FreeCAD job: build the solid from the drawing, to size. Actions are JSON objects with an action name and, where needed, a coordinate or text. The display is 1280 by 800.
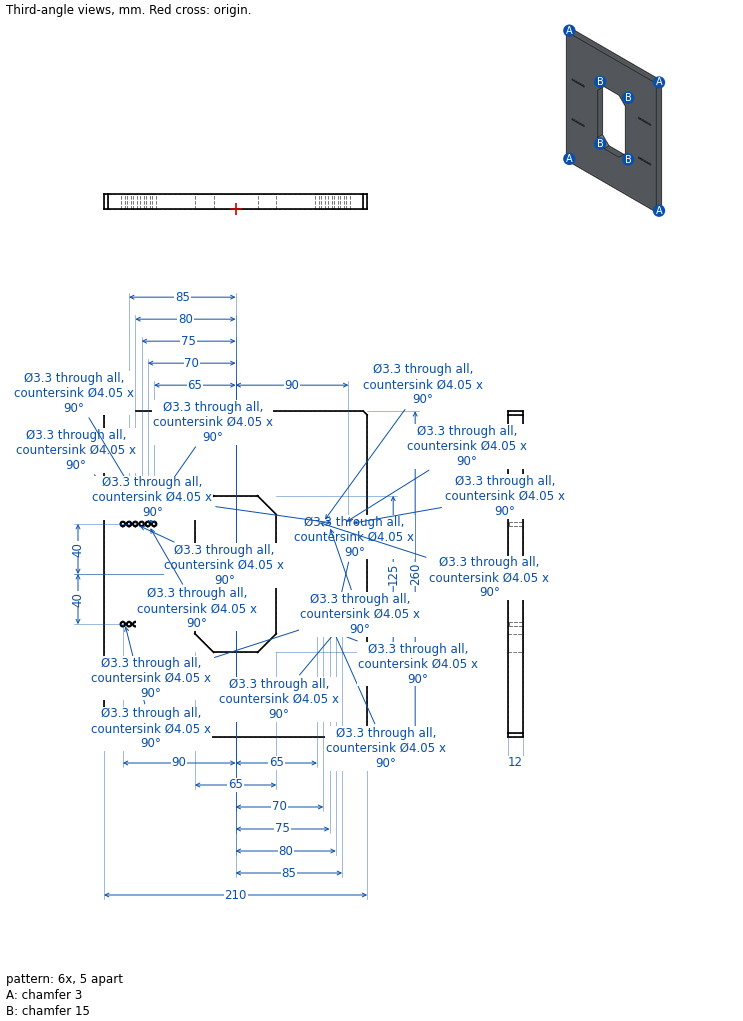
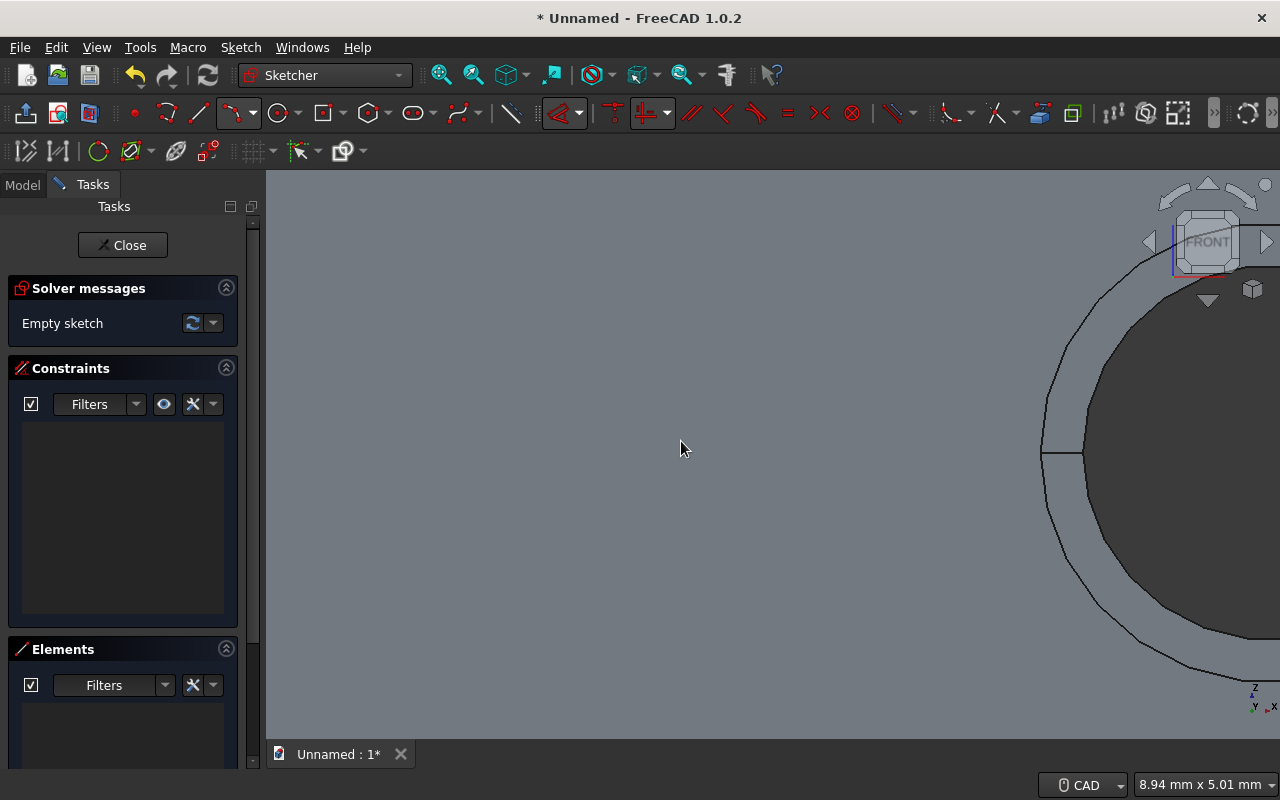
{"action": "left_click", "coordinate": [278, 114]}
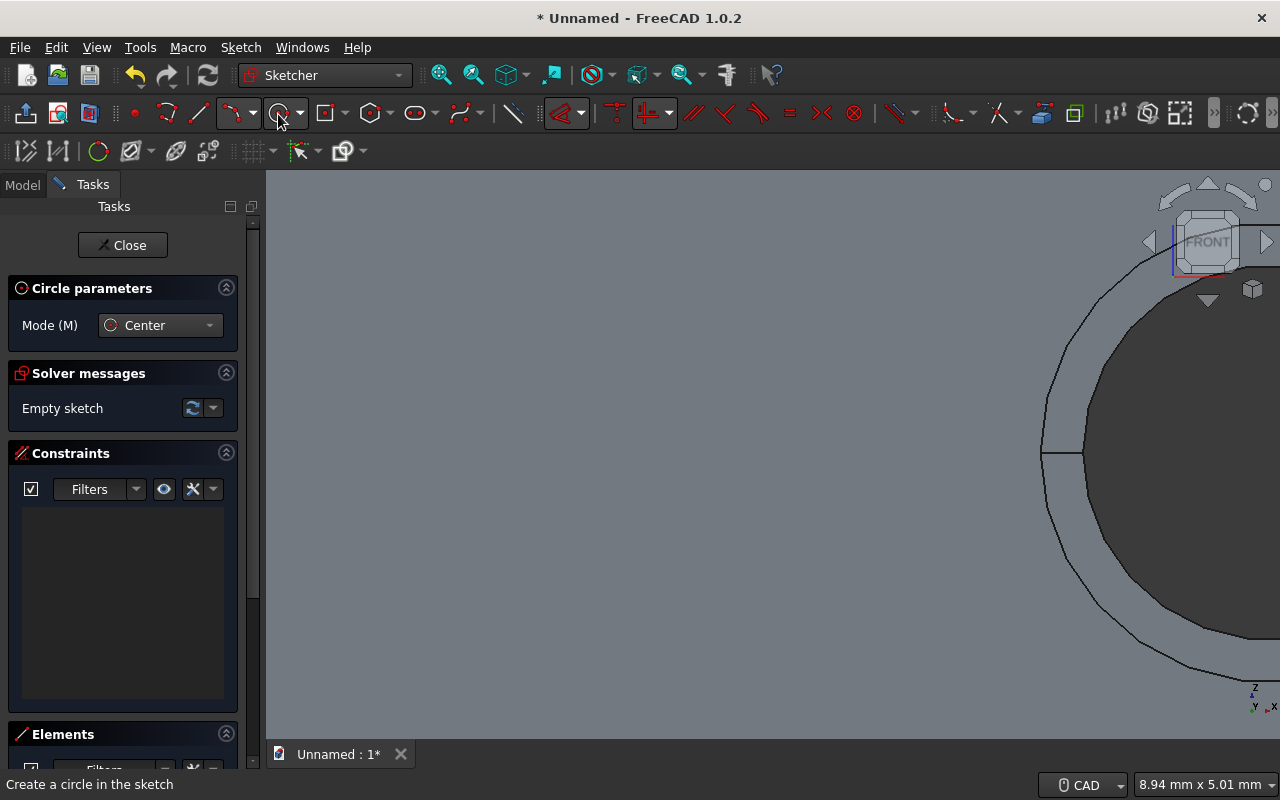
{"action": "left_click", "coordinate": [703, 453]}
{"action": "mouse_move", "coordinate": [835, 320]}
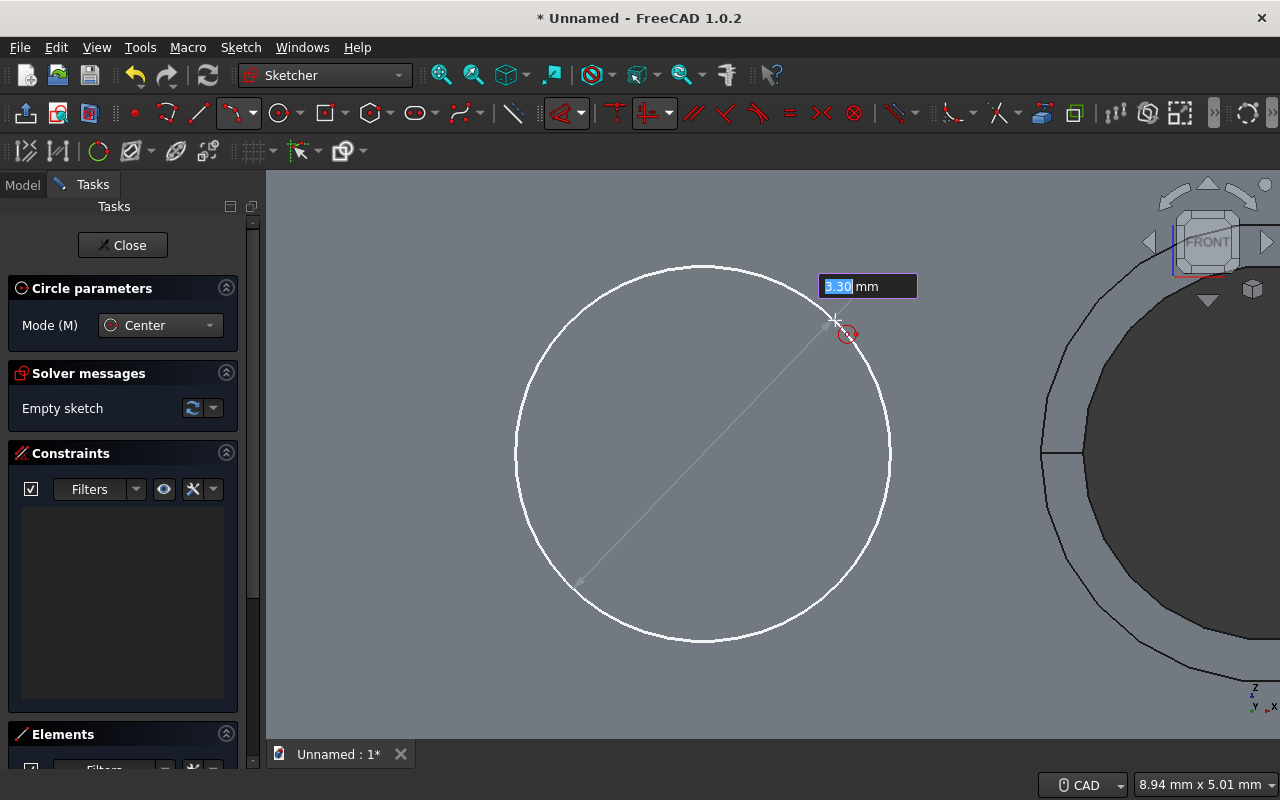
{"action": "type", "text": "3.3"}
{"action": "key", "text": "Return"}
{"action": "key", "text": "Escape"}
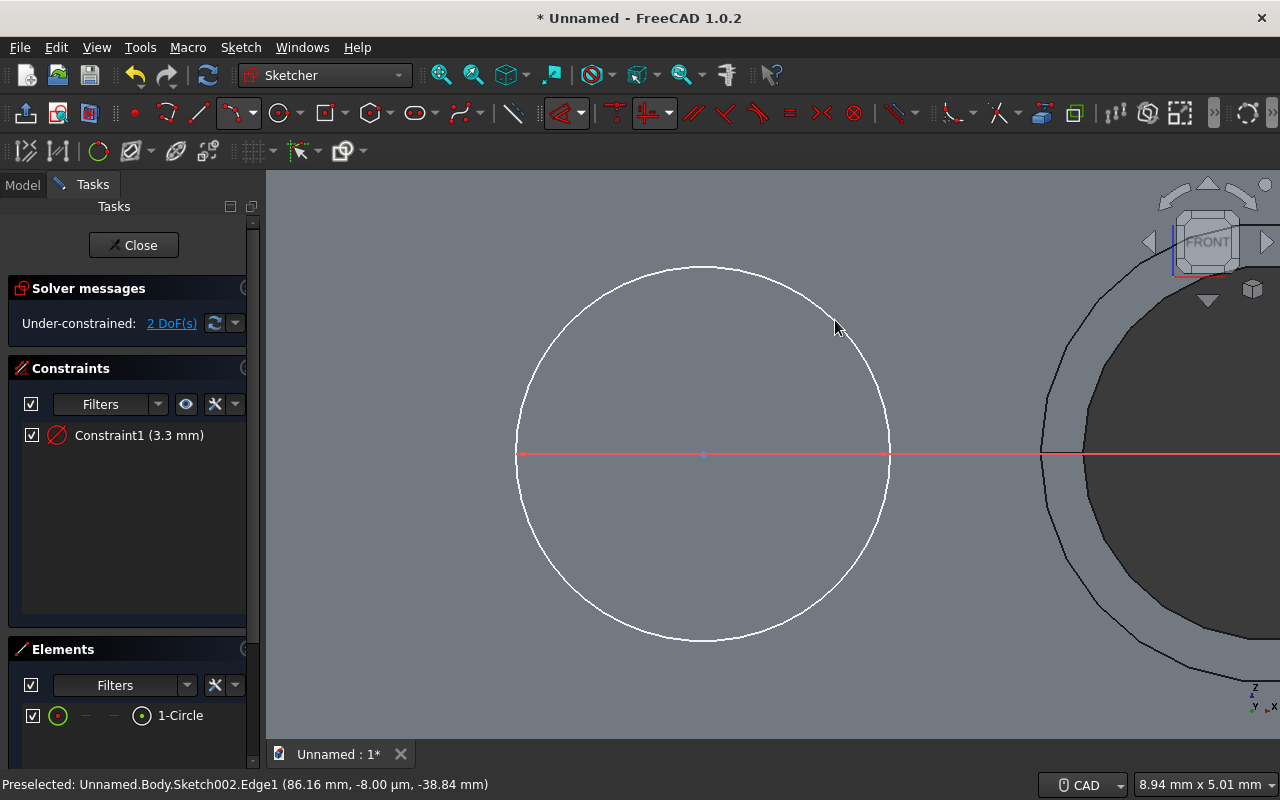
{"action": "left_click", "coordinate": [703, 454]}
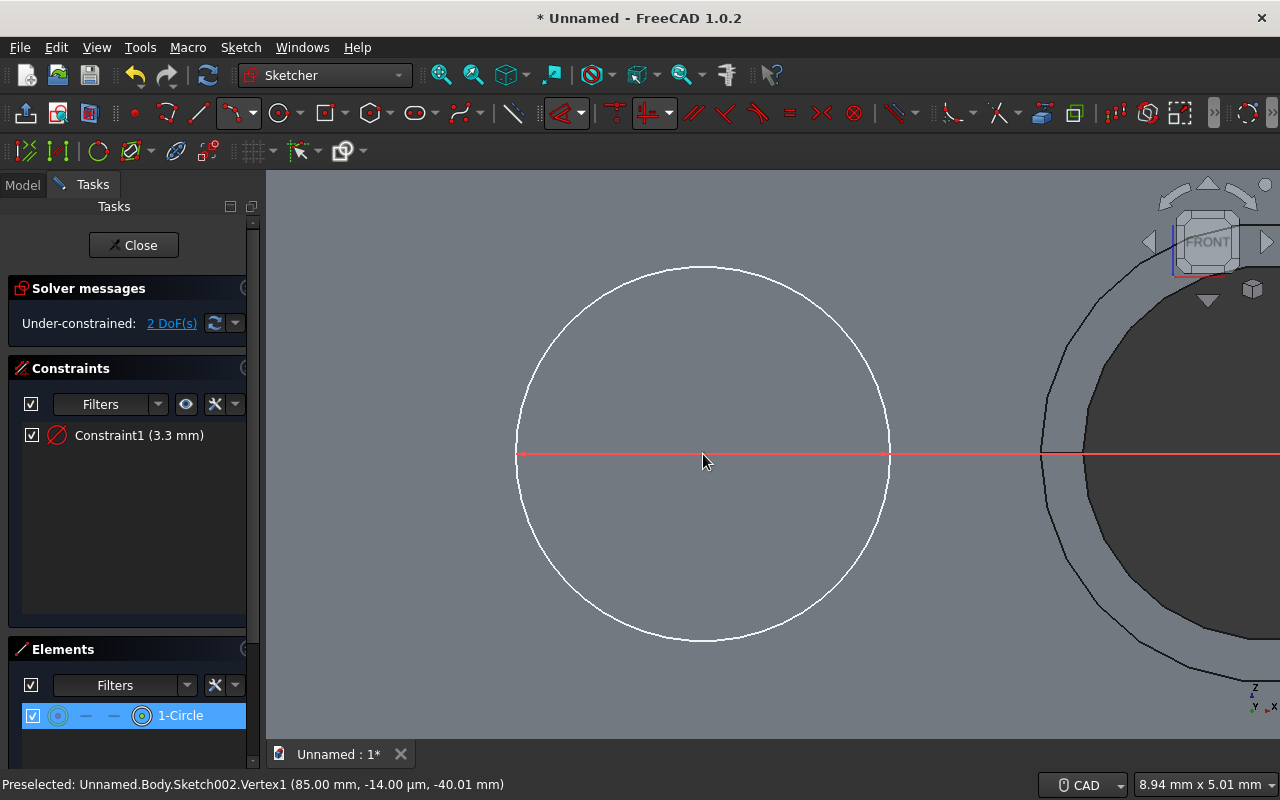
{"action": "left_click", "coordinate": [584, 114]}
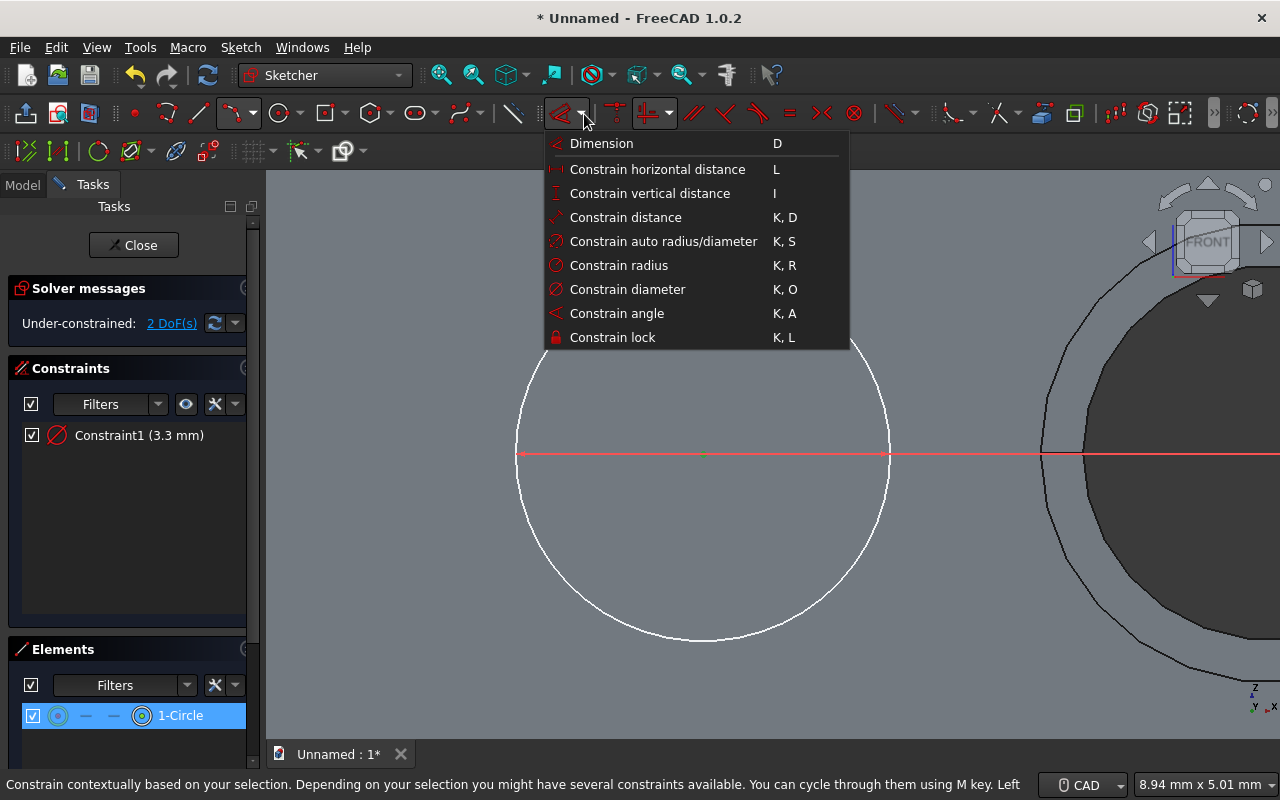
{"action": "left_click", "coordinate": [697, 169]}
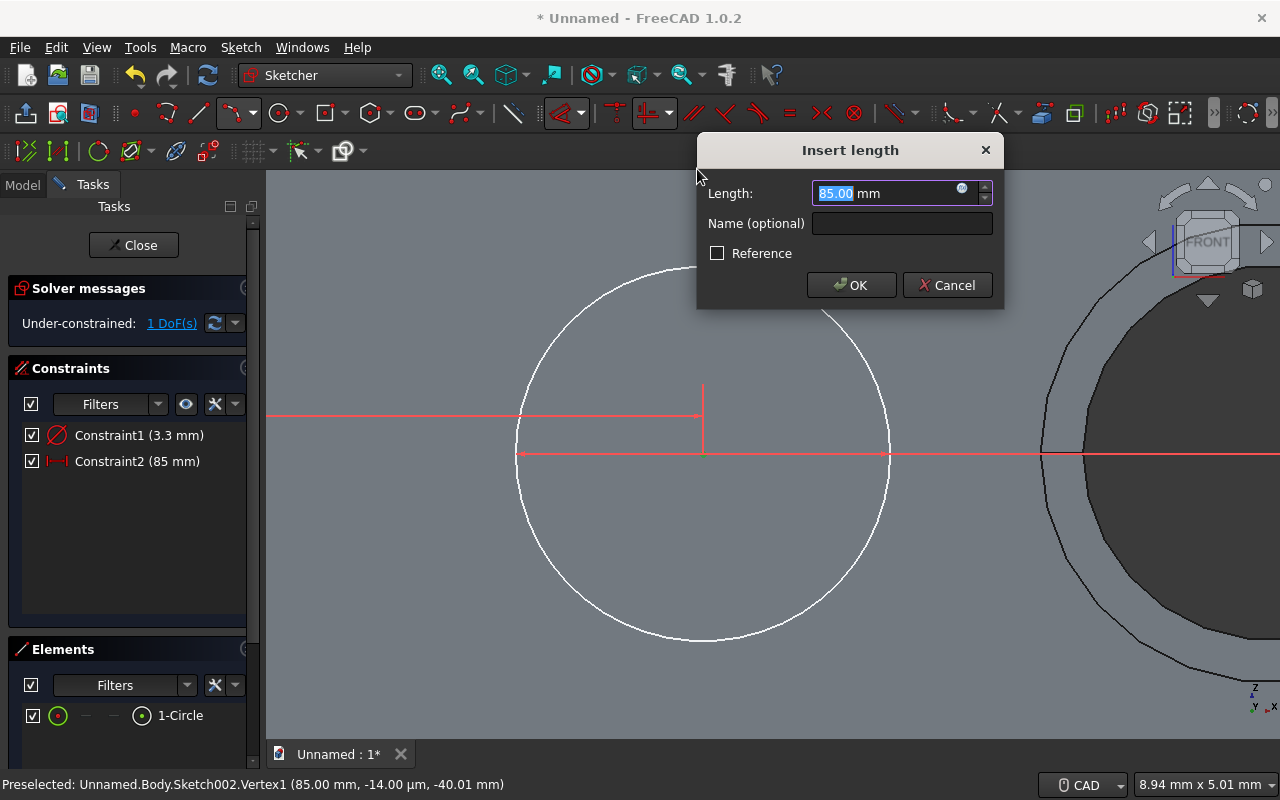
{"action": "type", "text": "85"}
{"action": "key", "text": "Return"}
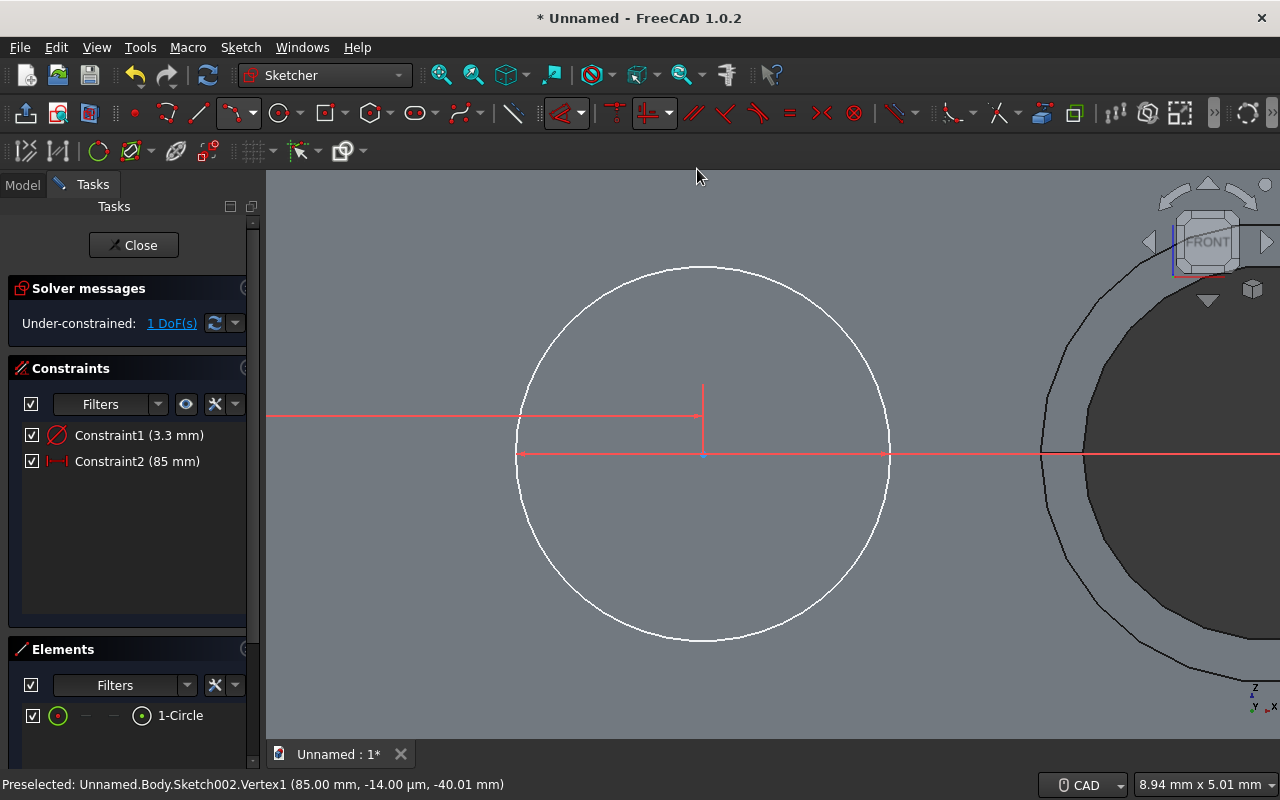
{"action": "left_click", "coordinate": [703, 454]}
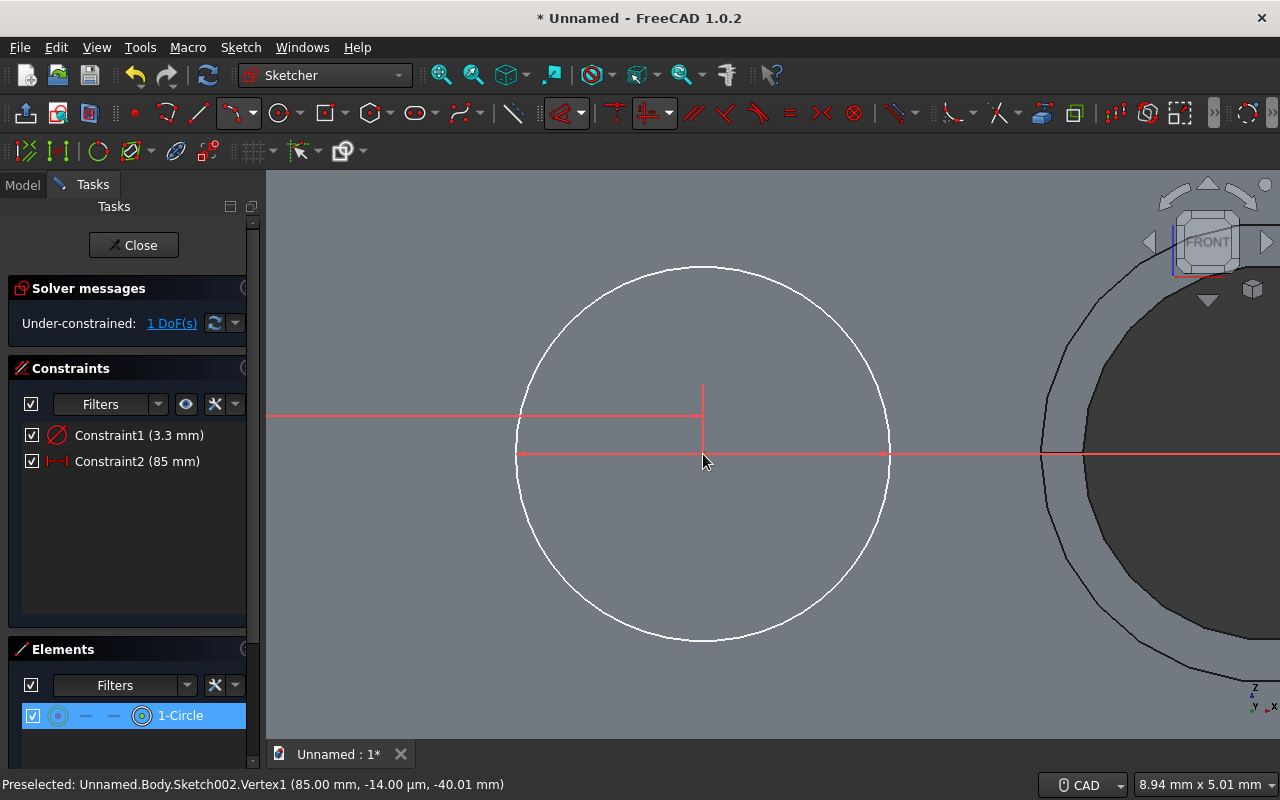
{"action": "key", "text": "i"}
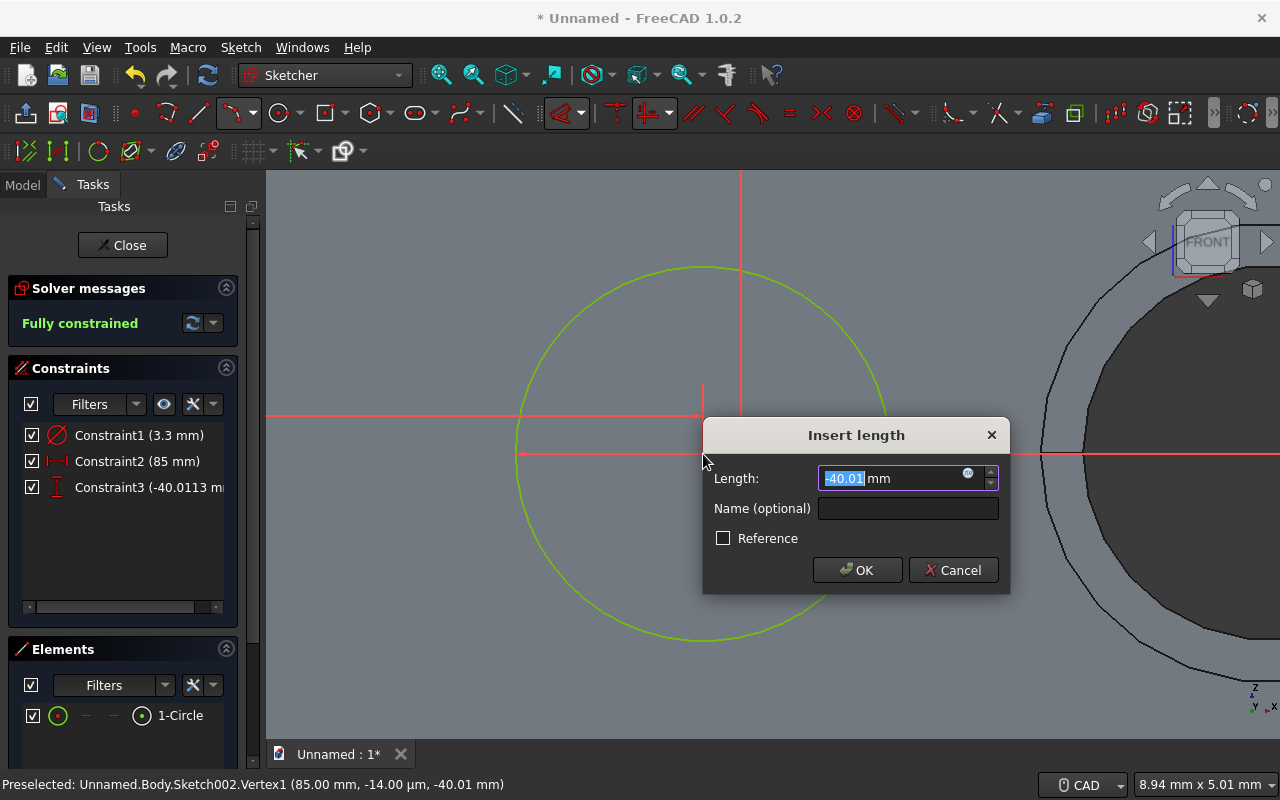
{"action": "type", "text": "-40"}
{"action": "key", "text": "Return"}